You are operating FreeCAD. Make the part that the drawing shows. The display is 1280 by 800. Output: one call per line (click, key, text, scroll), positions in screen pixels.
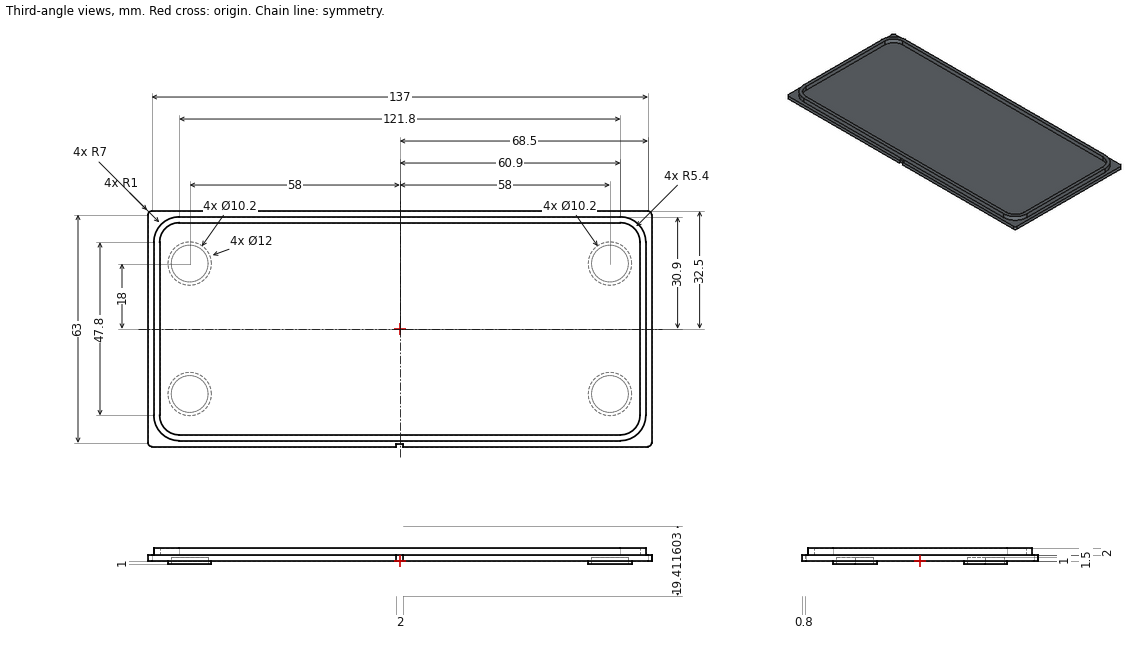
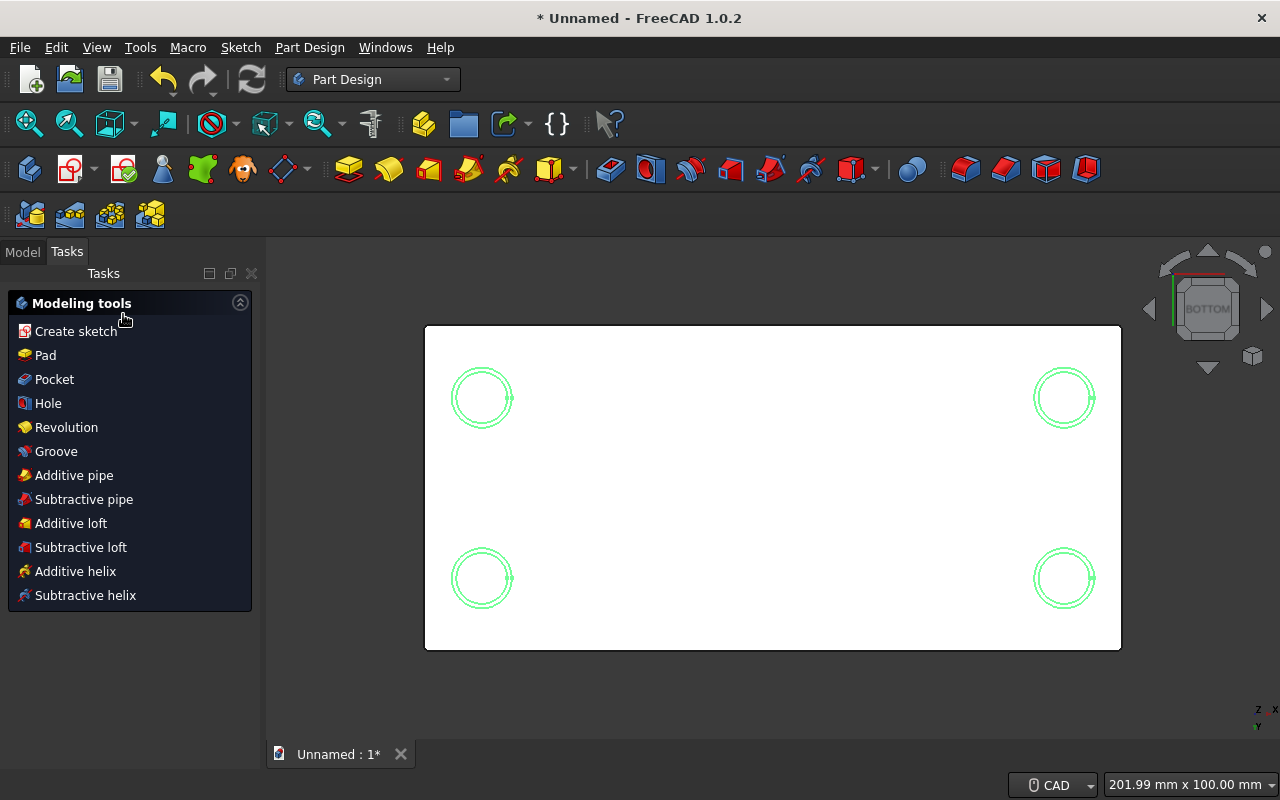
click(350, 170)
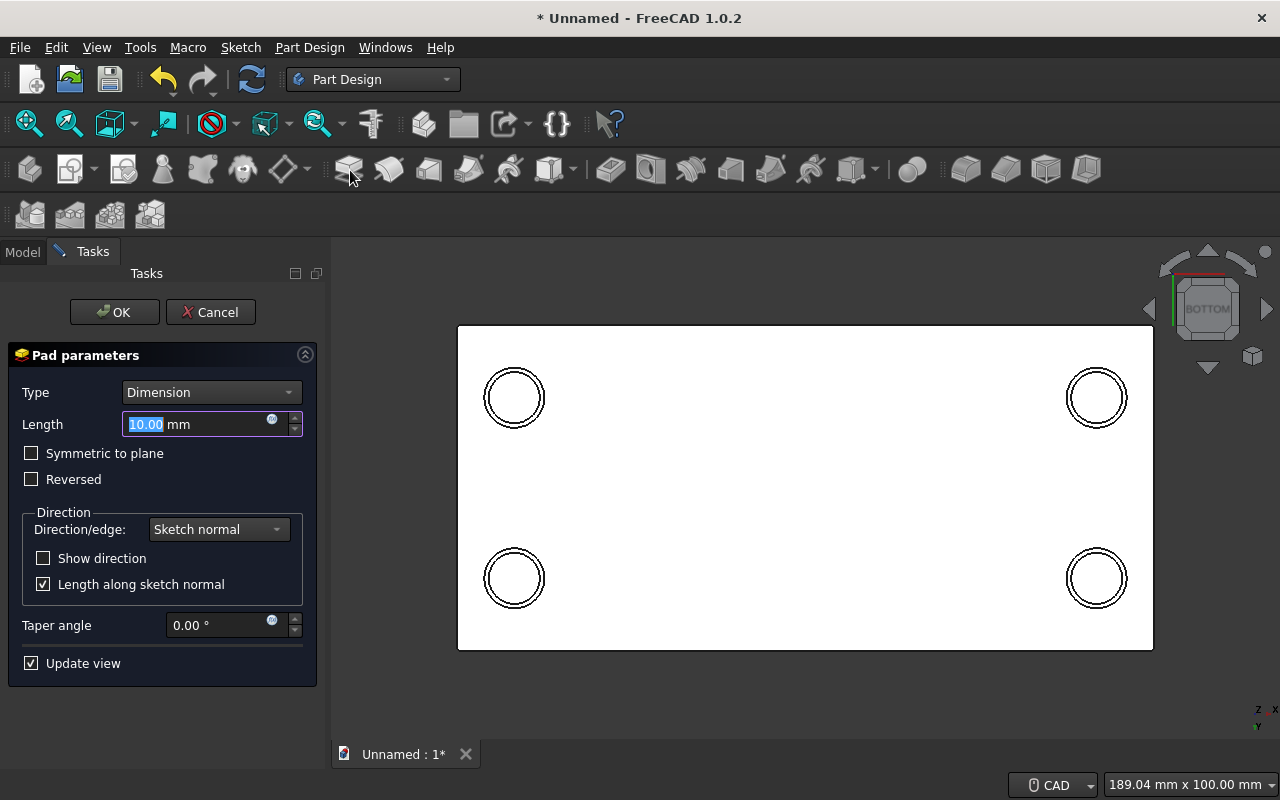
text(1)
key(Tab)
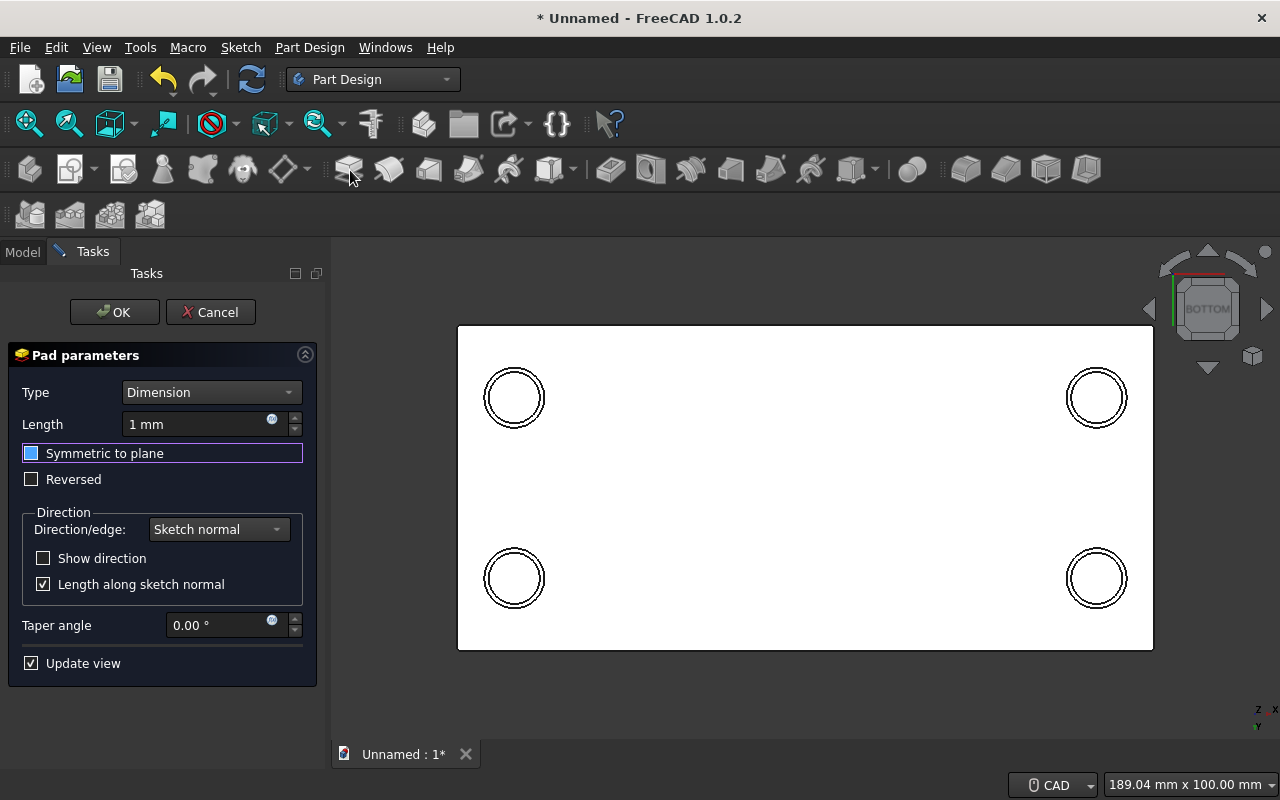
click(115, 312)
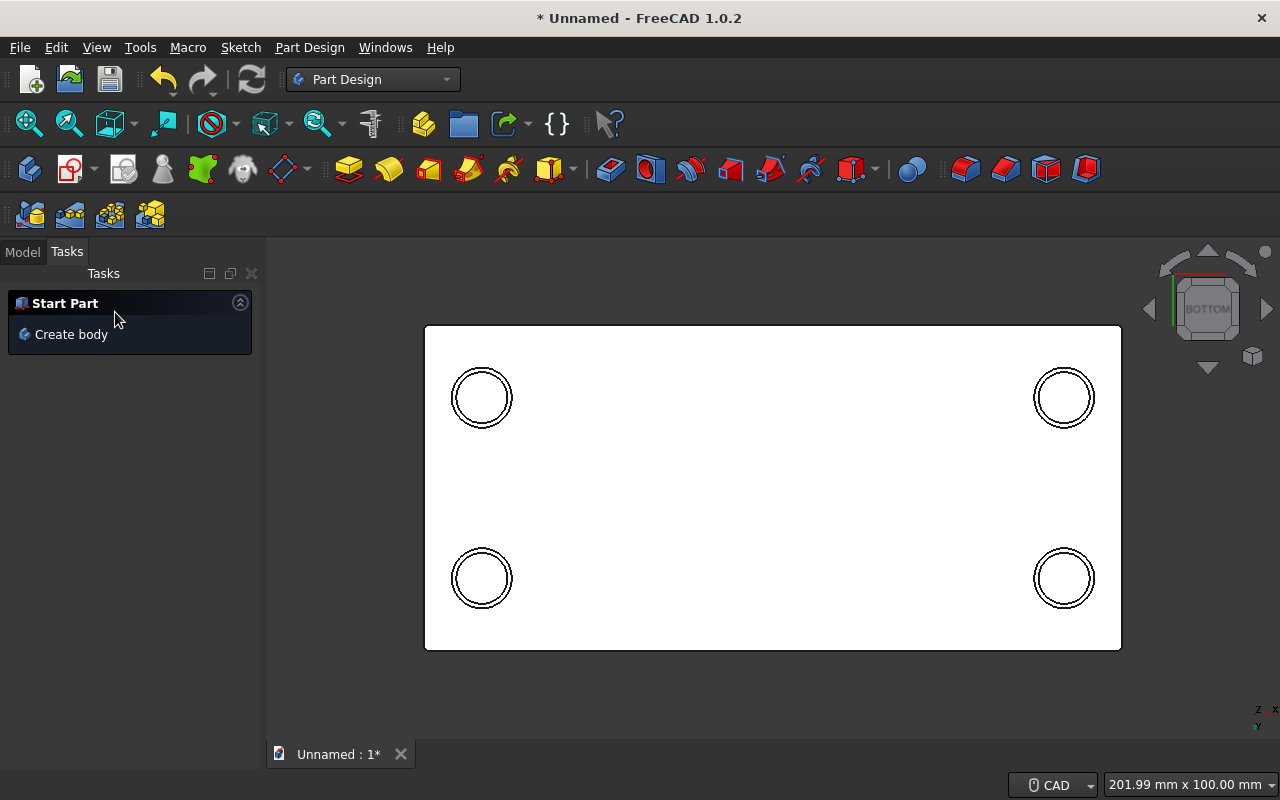
key(0)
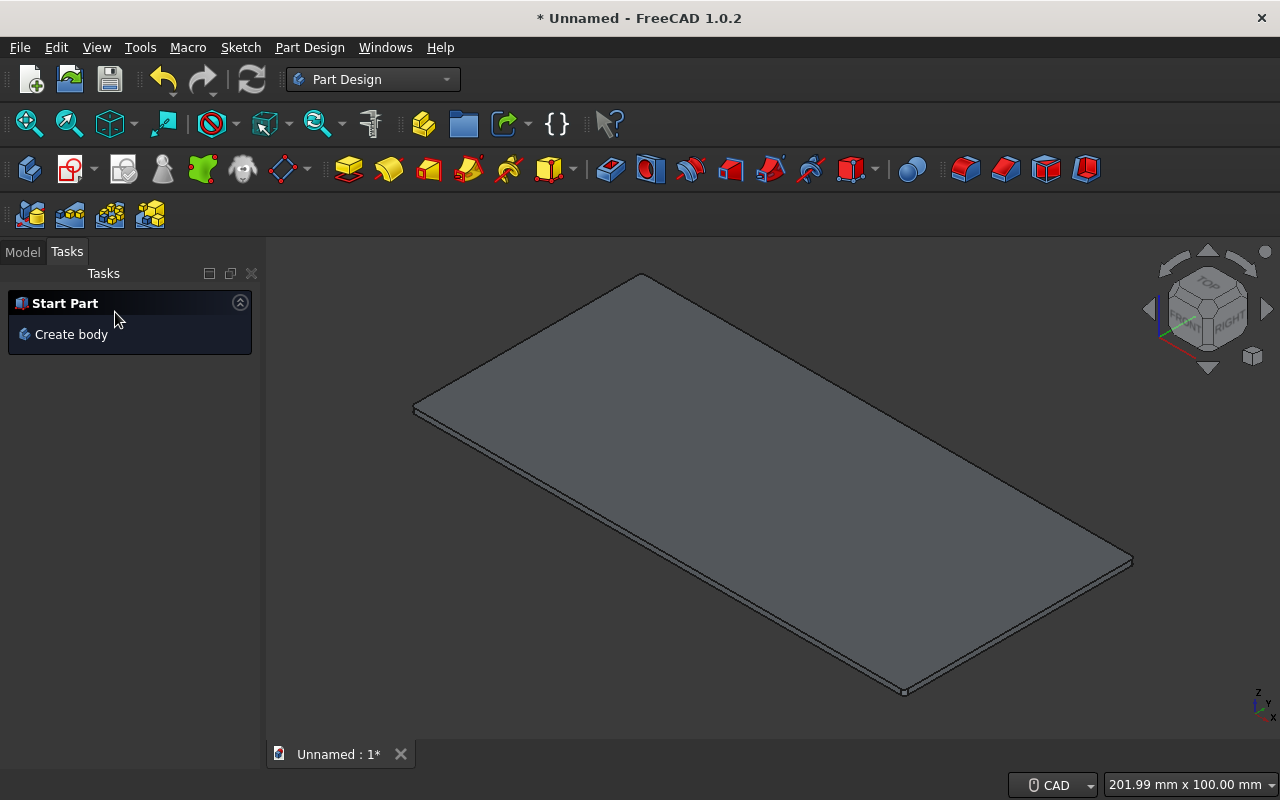
click(843, 522)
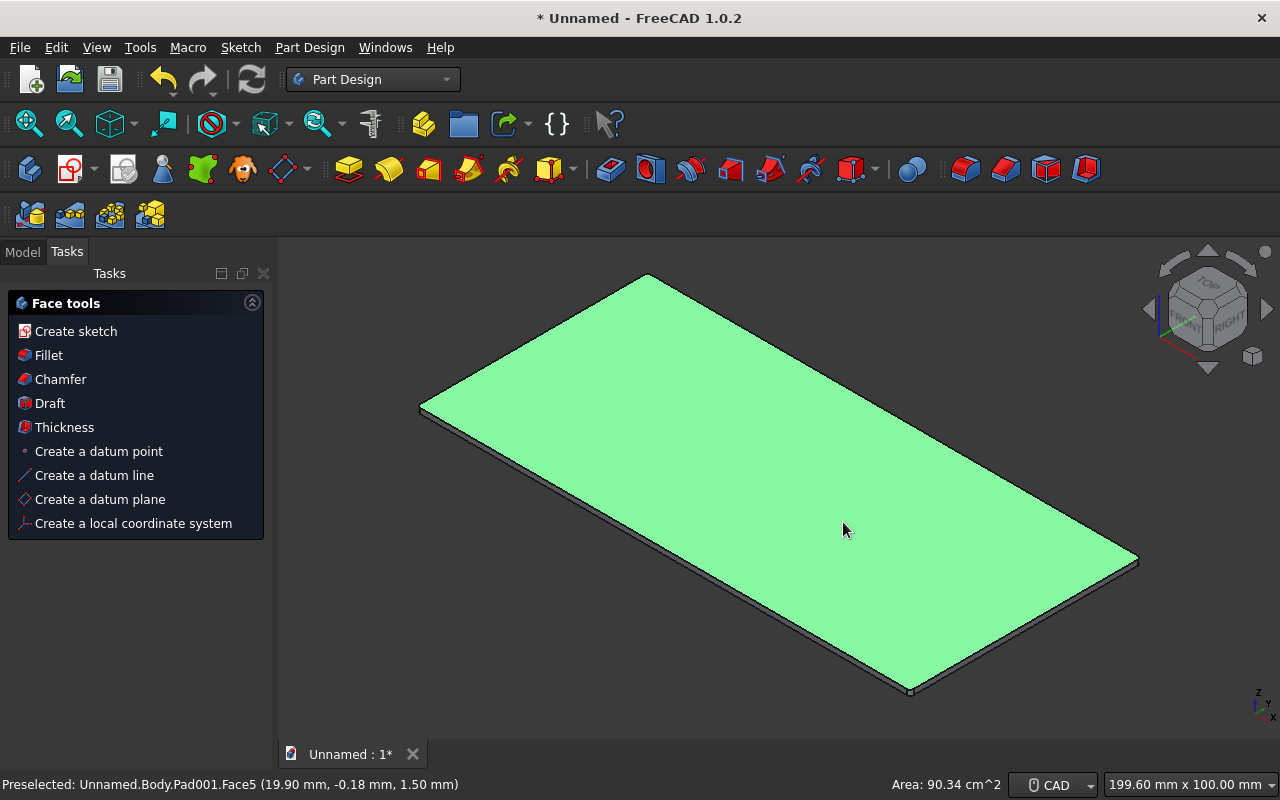
click(70, 170)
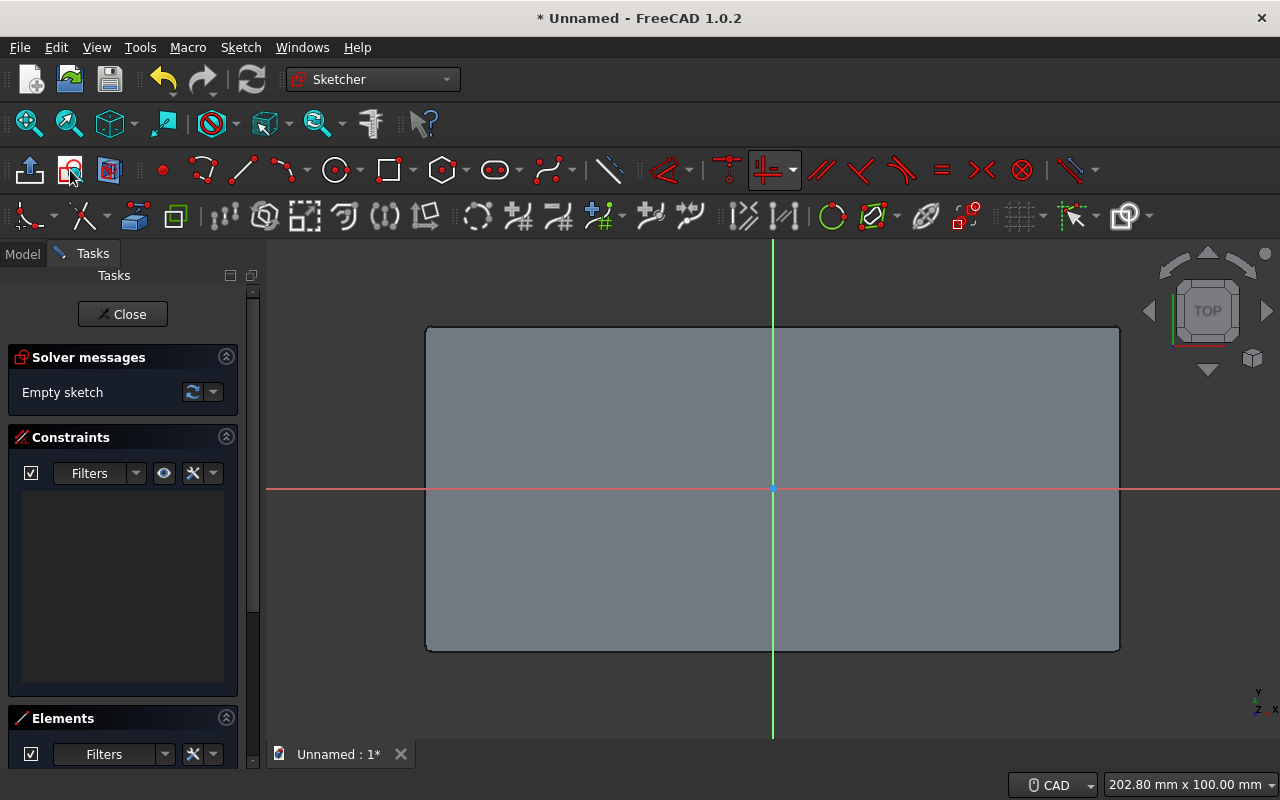
scroll(395, 489, down, 1)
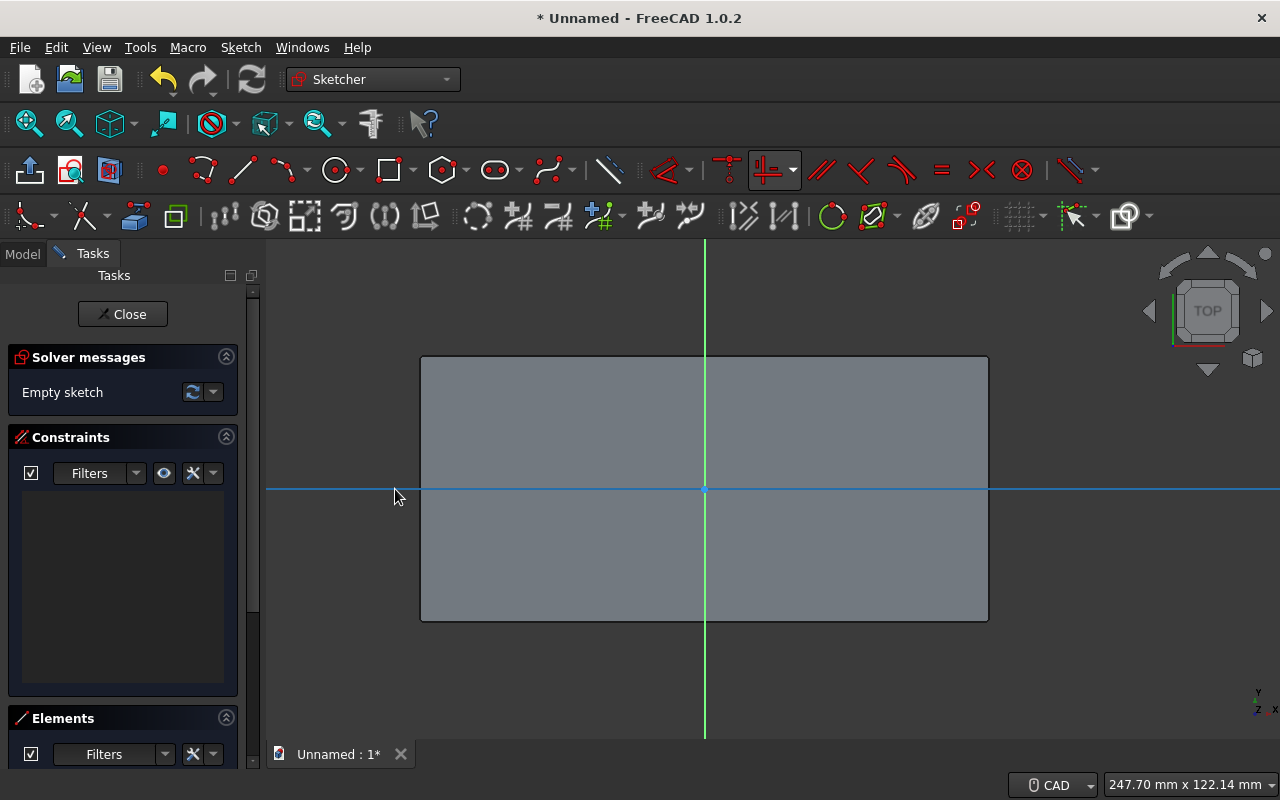
click(244, 170)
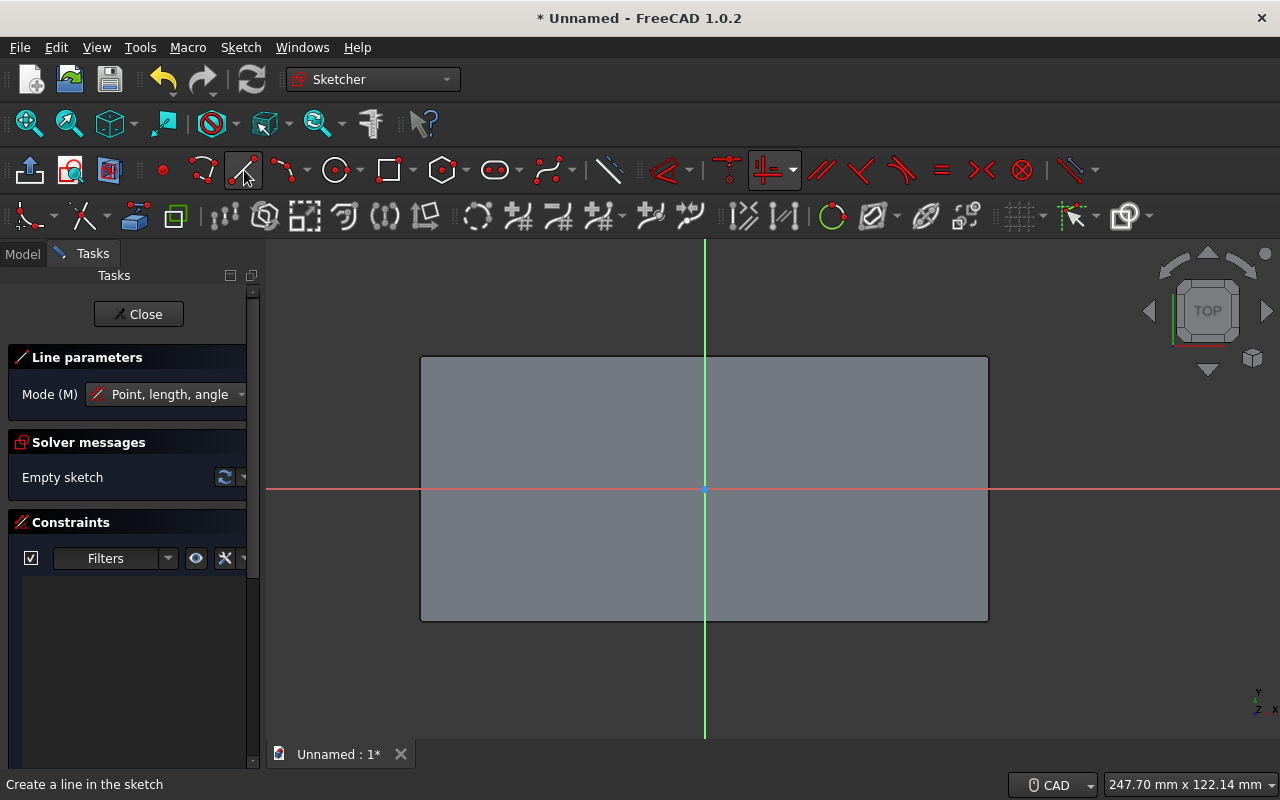
click(954, 363)
click(455, 363)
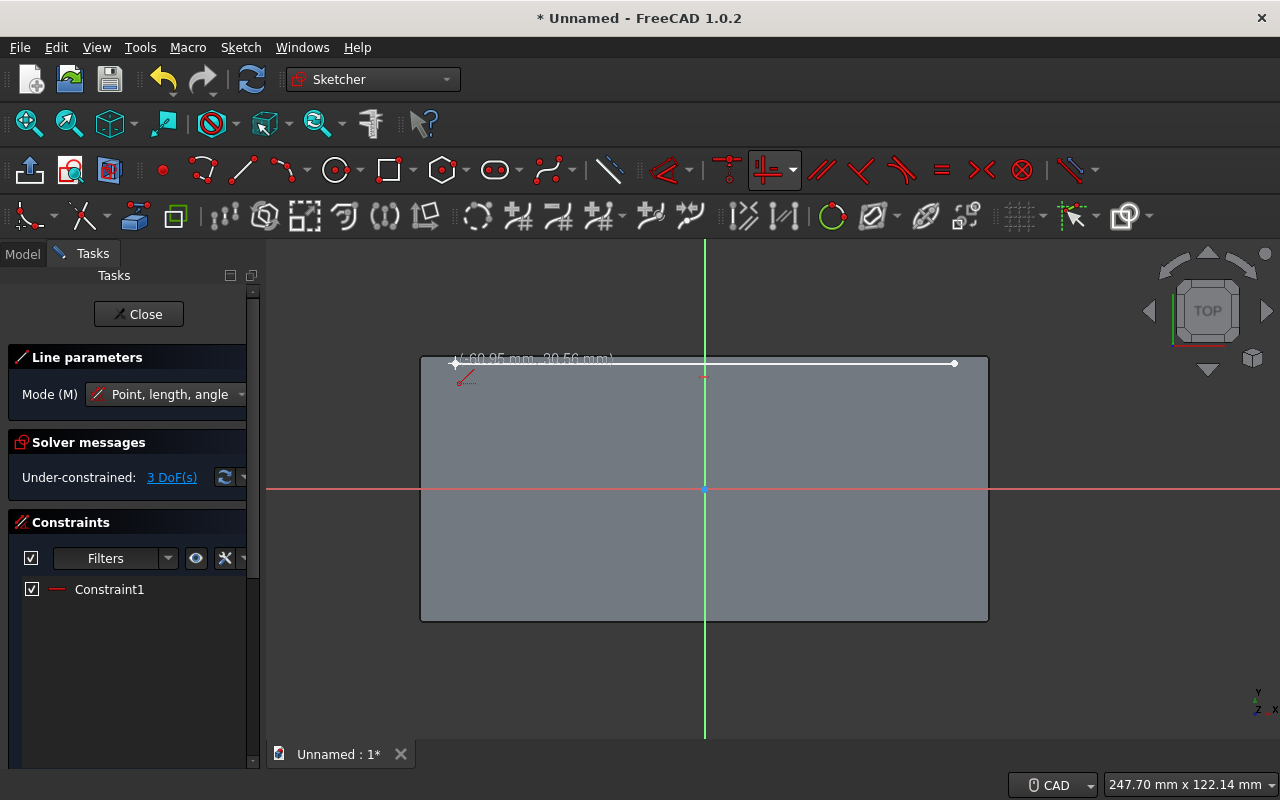
click(427, 391)
click(427, 587)